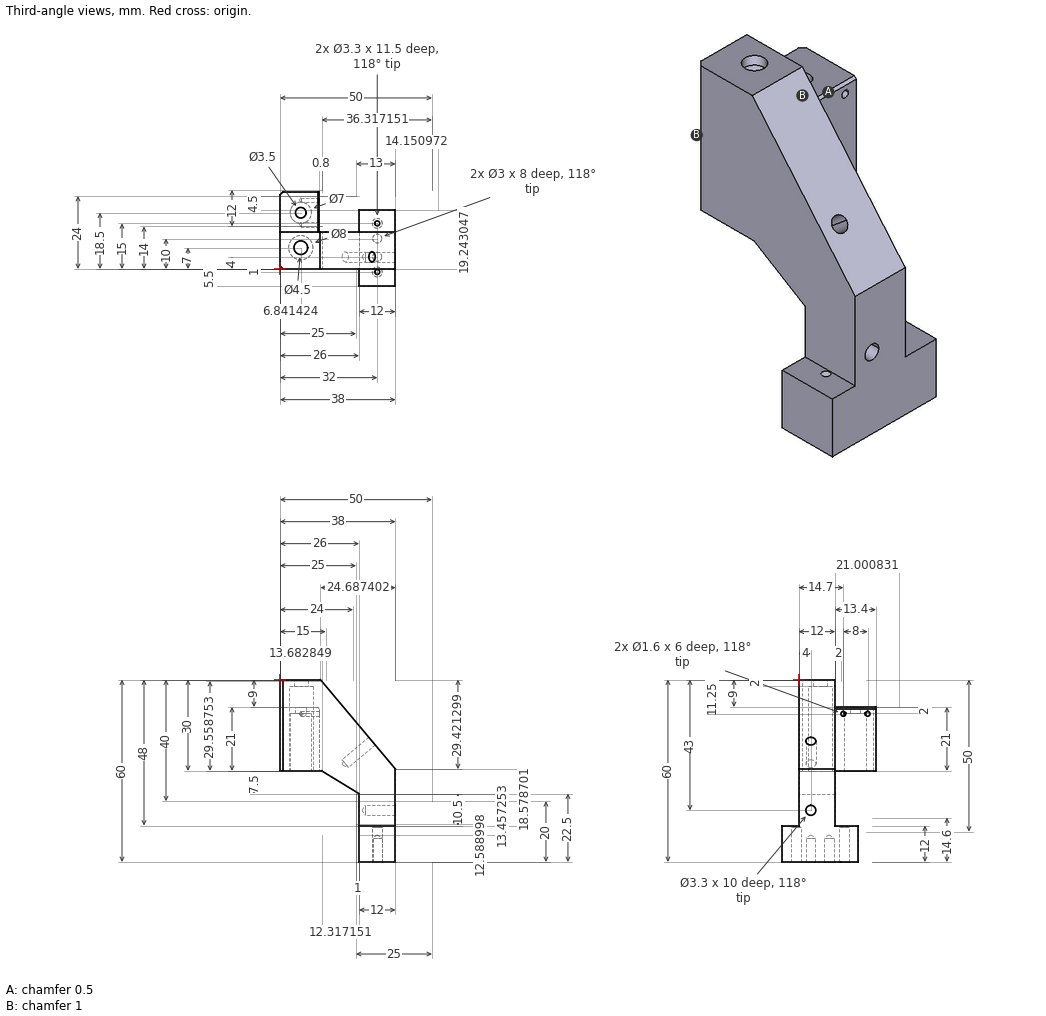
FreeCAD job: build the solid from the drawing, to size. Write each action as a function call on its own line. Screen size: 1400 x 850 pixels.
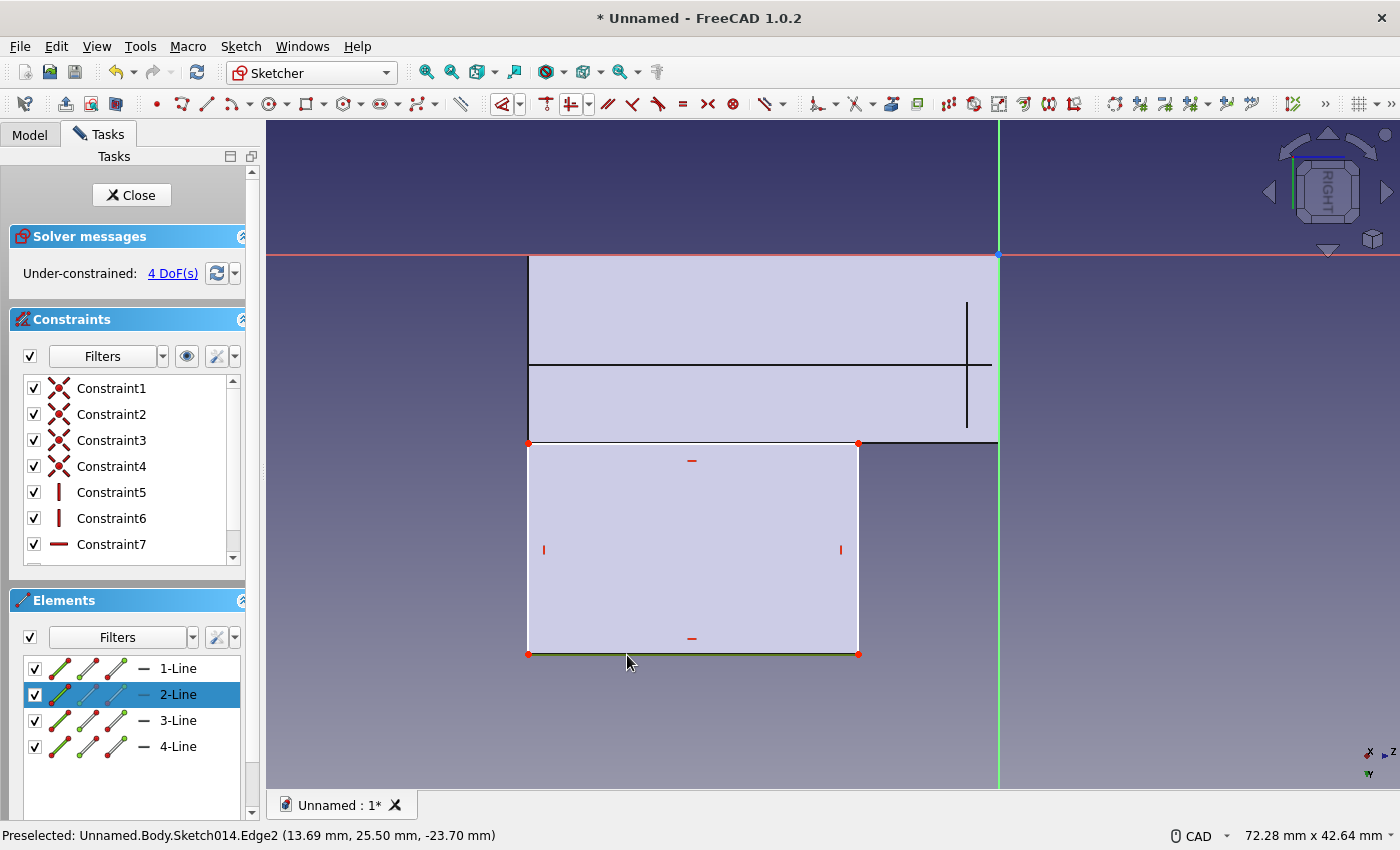
key(l)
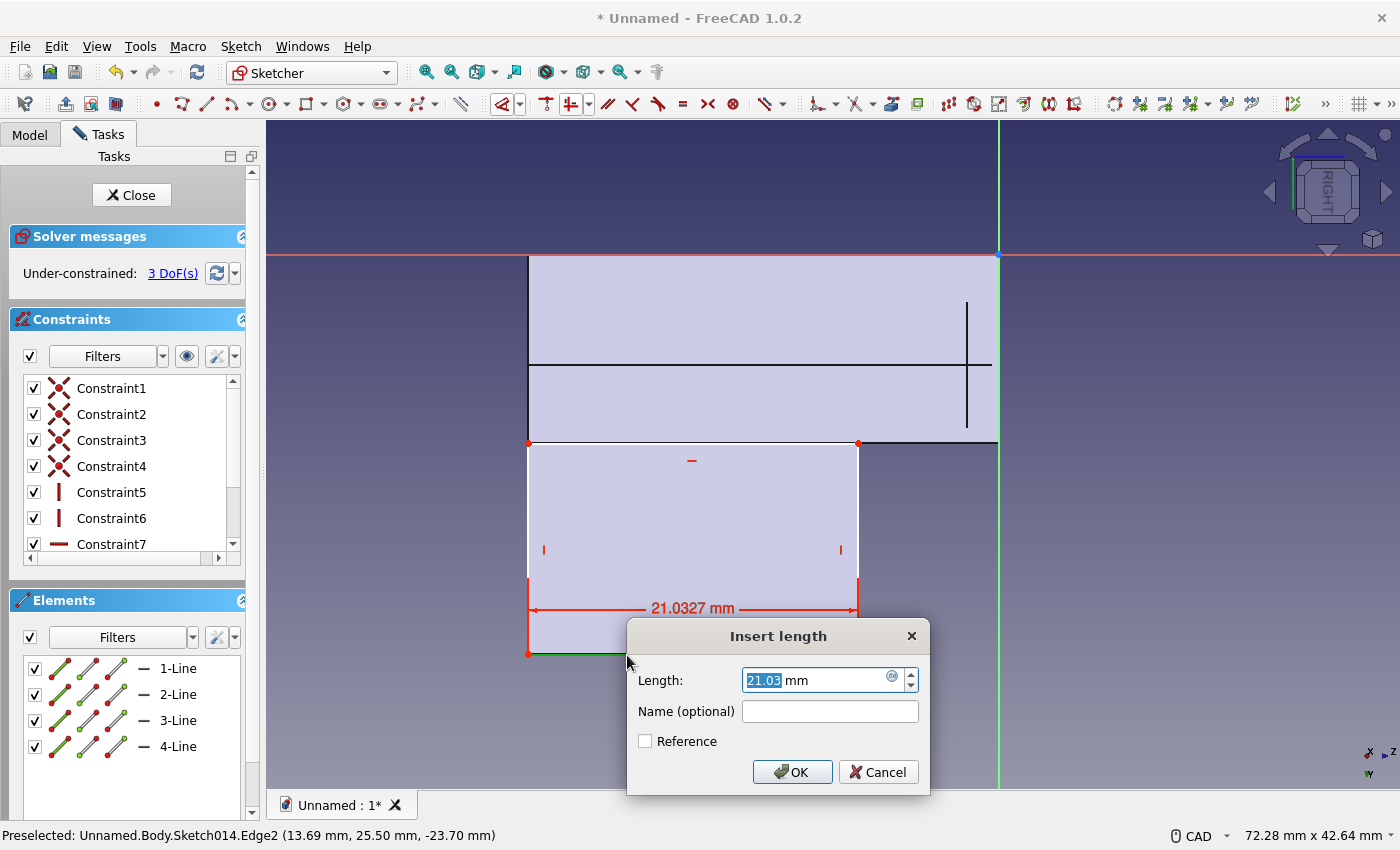
text(21)
key(Return)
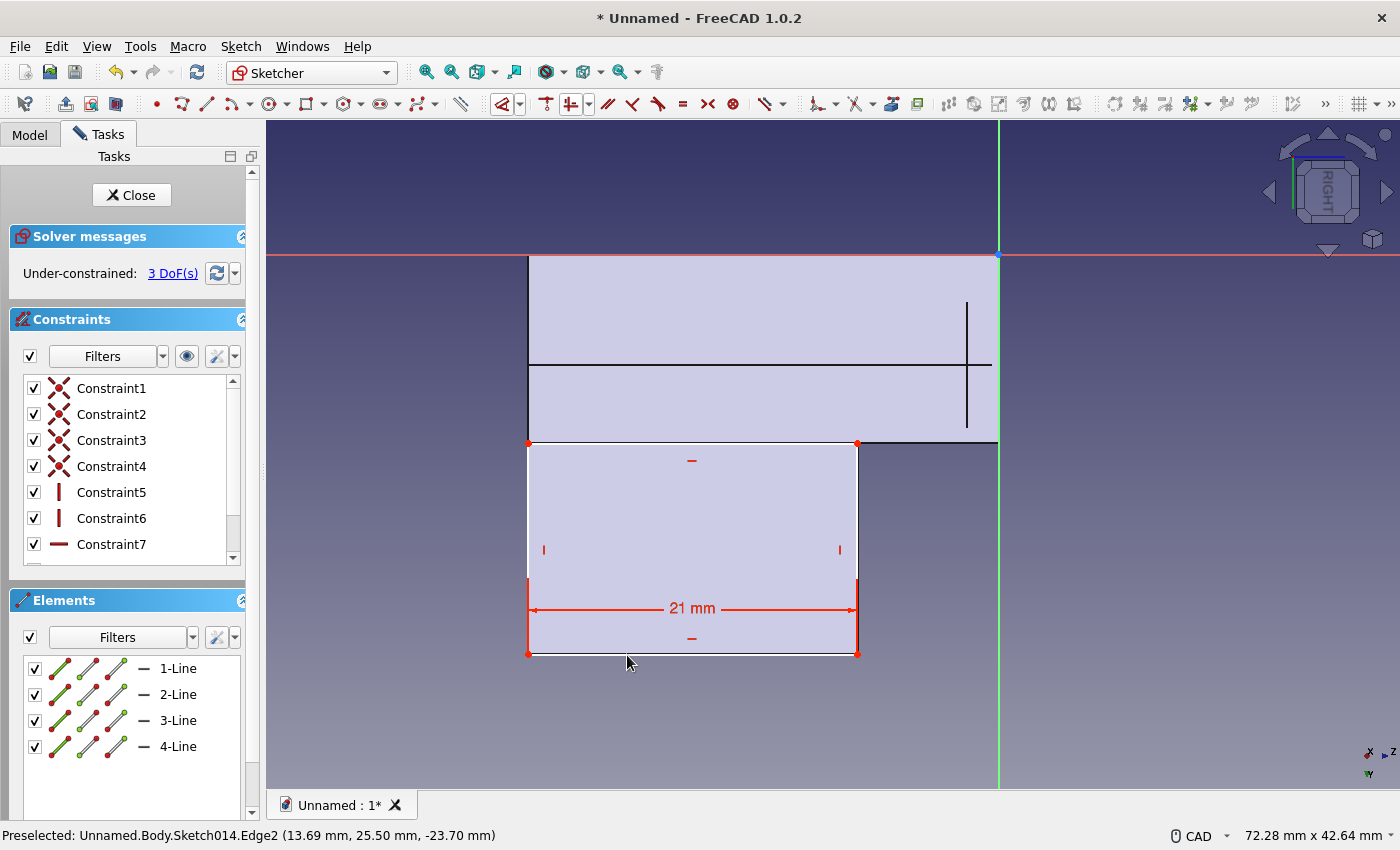
click(857, 655)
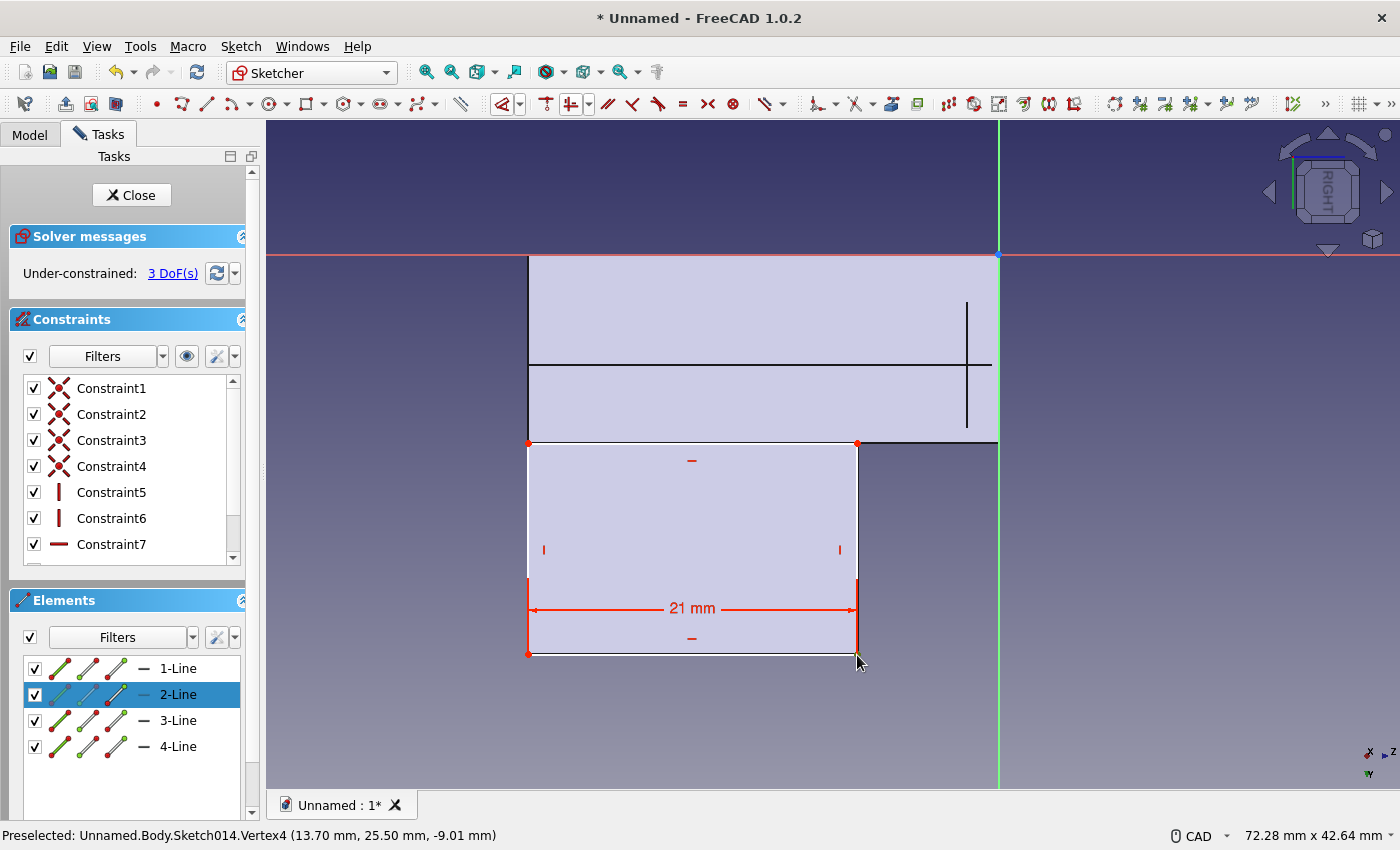
key(l)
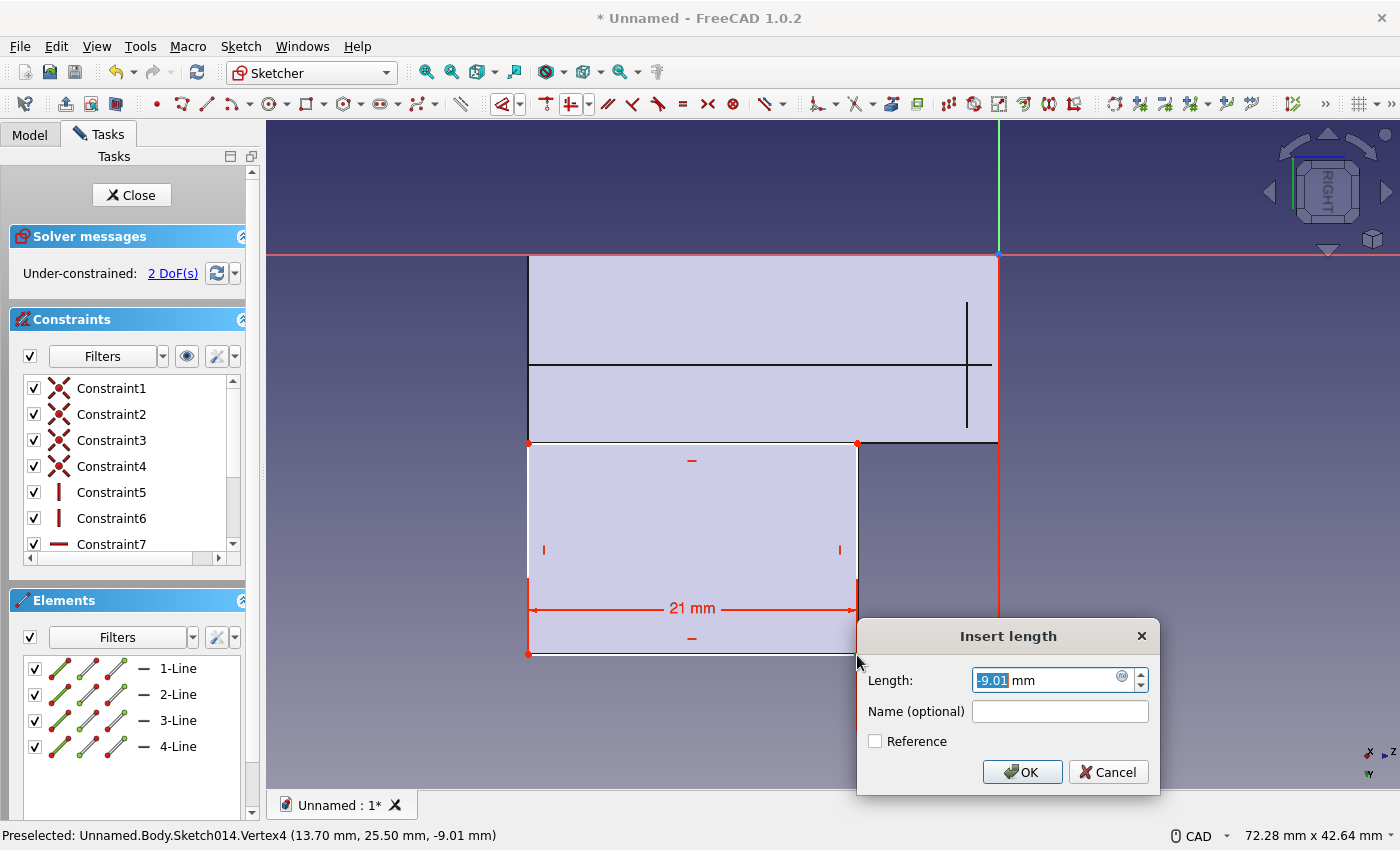
text(-9)
key(Return)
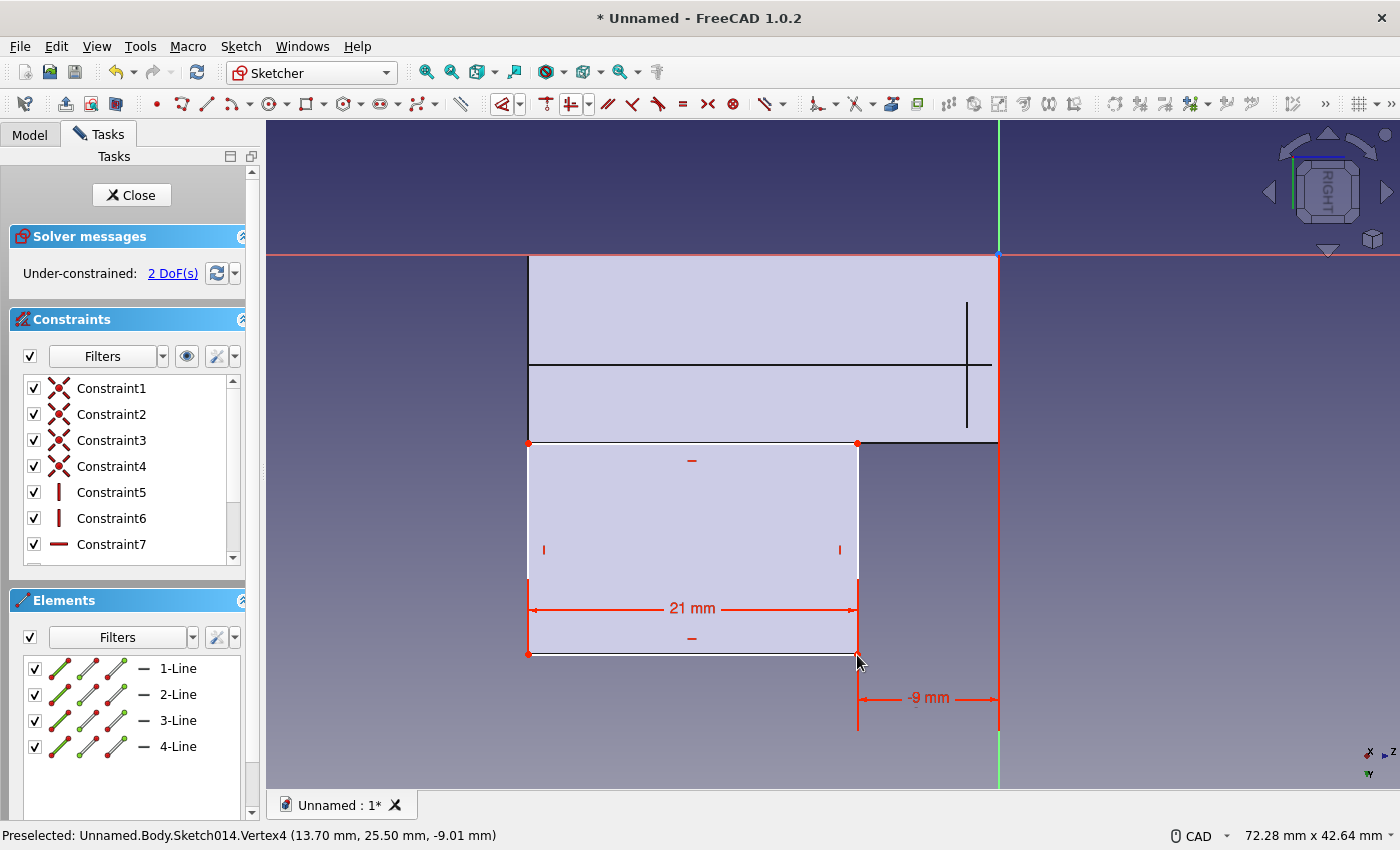
click(528, 444)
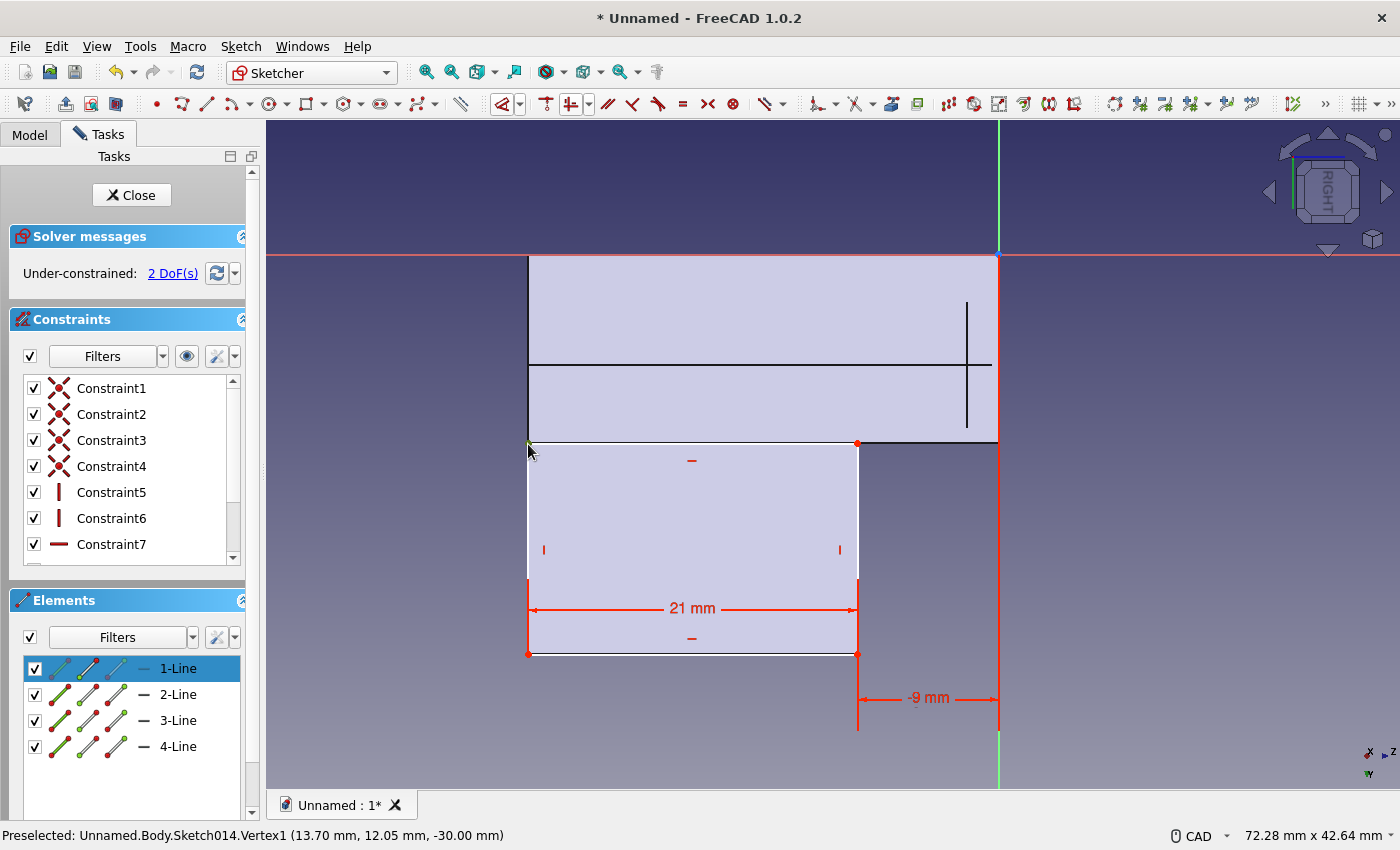
key(i)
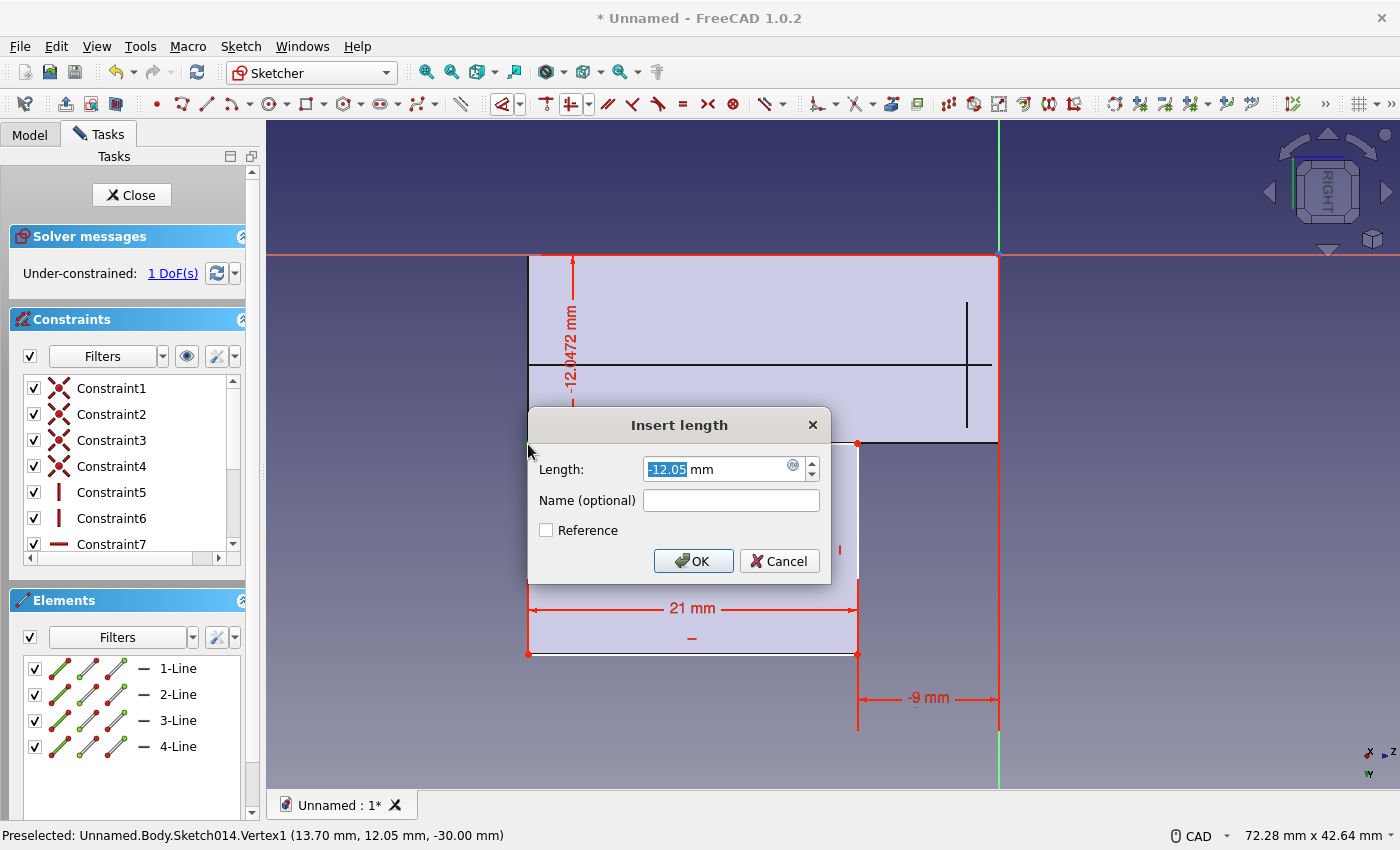
text(-12)
key(Return)